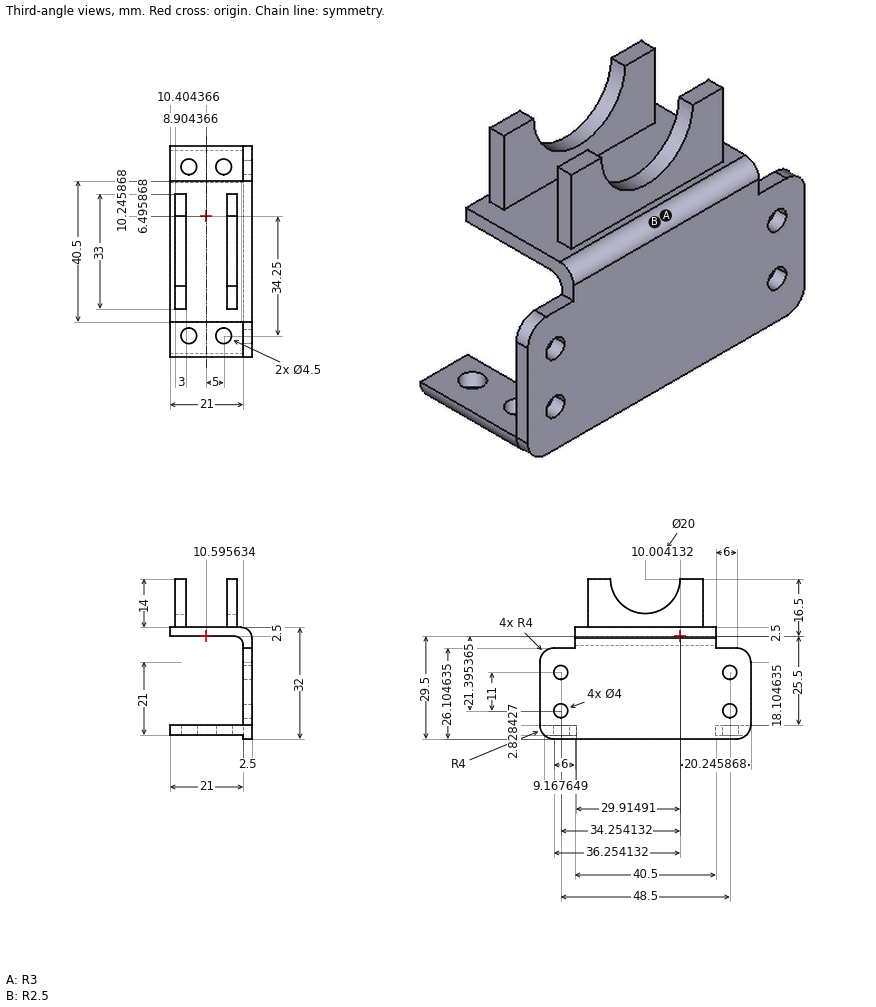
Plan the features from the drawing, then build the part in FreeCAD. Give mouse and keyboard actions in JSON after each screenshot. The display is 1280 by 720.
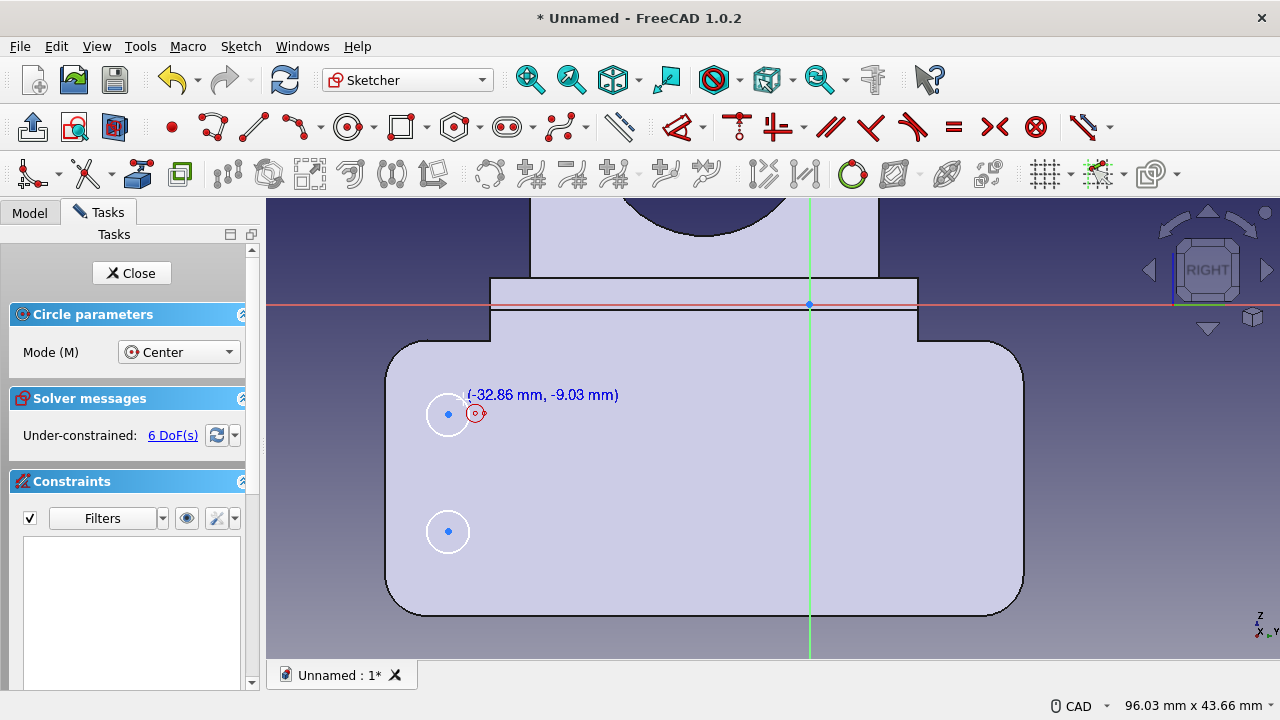
{"action": "left_click", "coordinate": [960, 414]}
{"action": "left_click", "coordinate": [975, 399]}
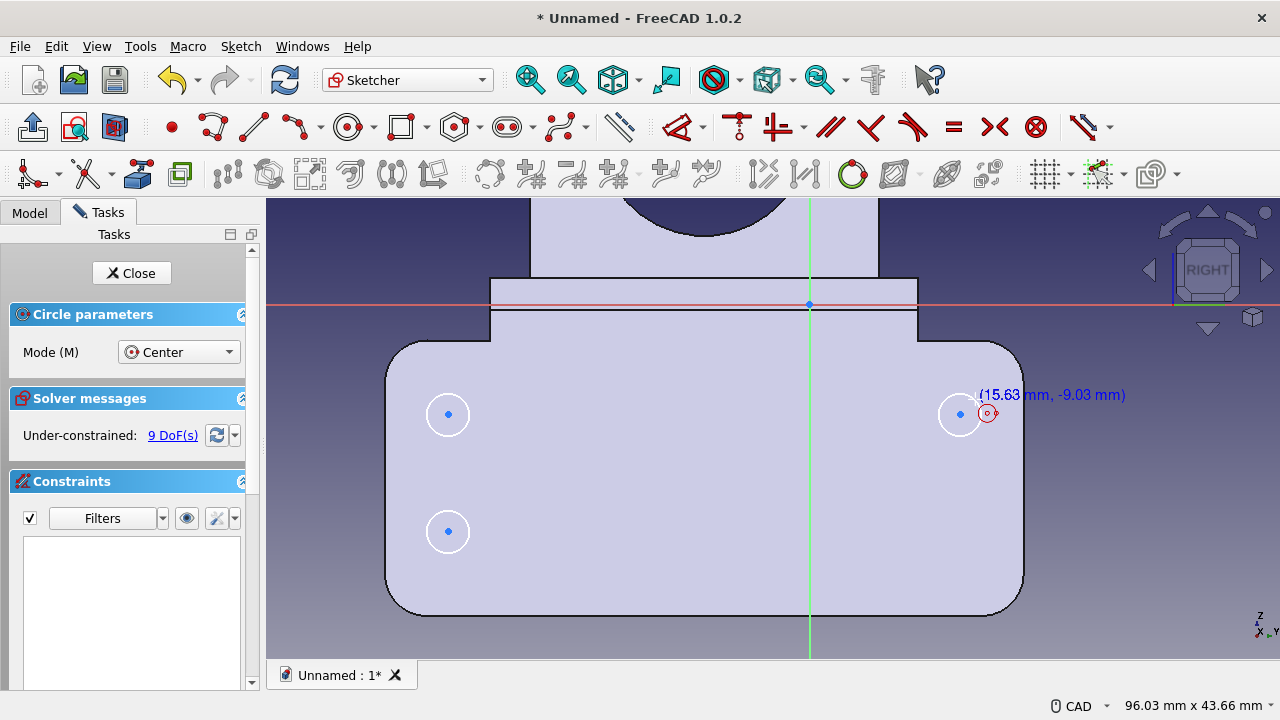
{"action": "left_click", "coordinate": [960, 531]}
{"action": "left_click", "coordinate": [975, 516]}
{"action": "key", "text": "Escape"}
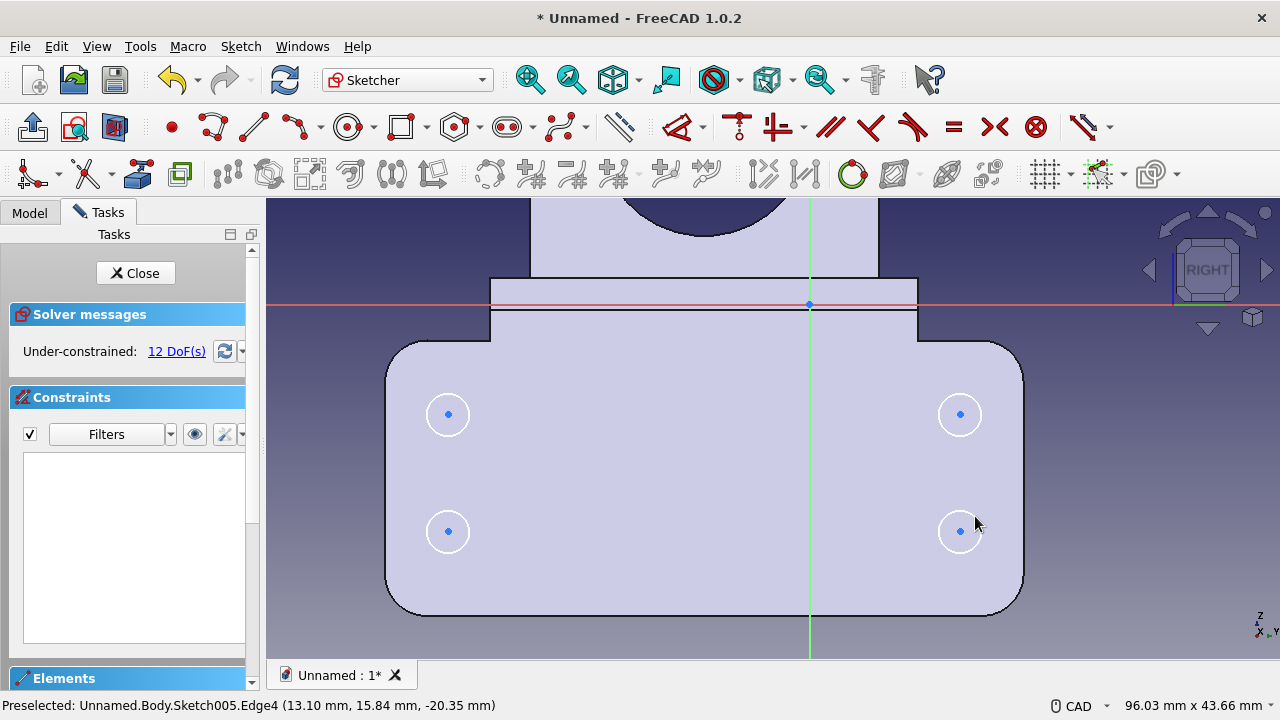
{"action": "left_click", "coordinate": [463, 517]}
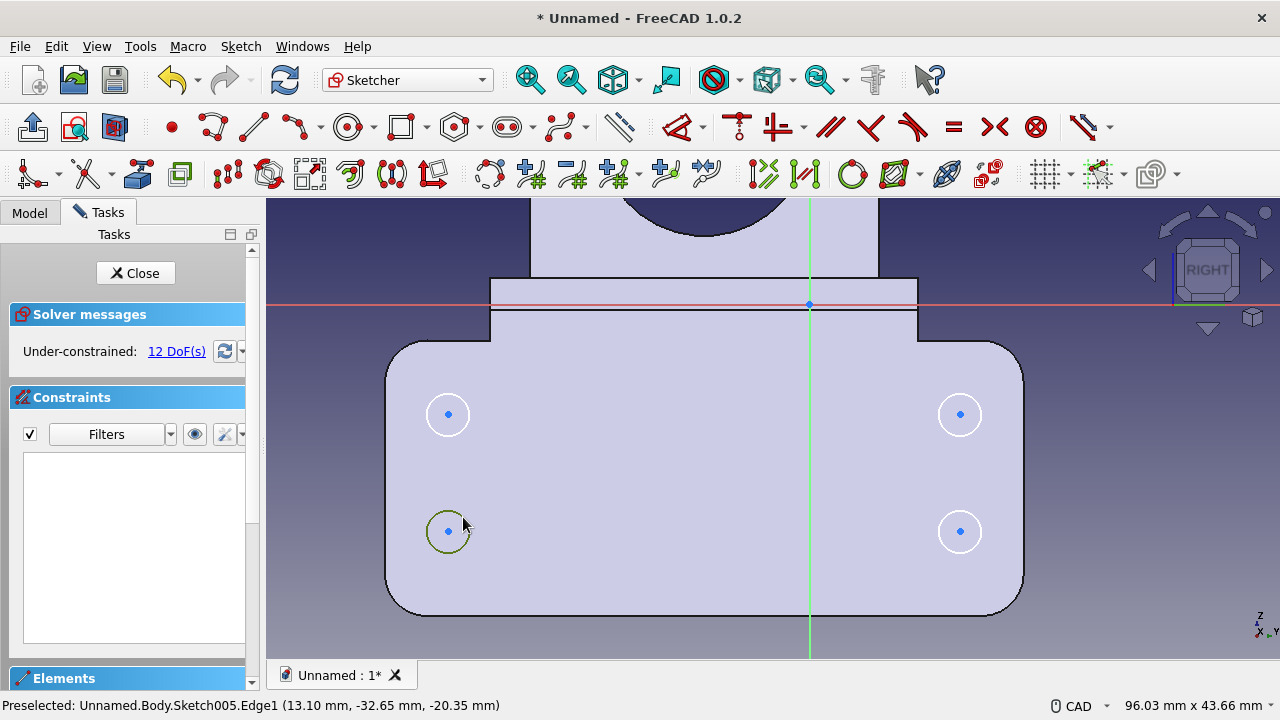
{"action": "left_click", "coordinate": [463, 400]}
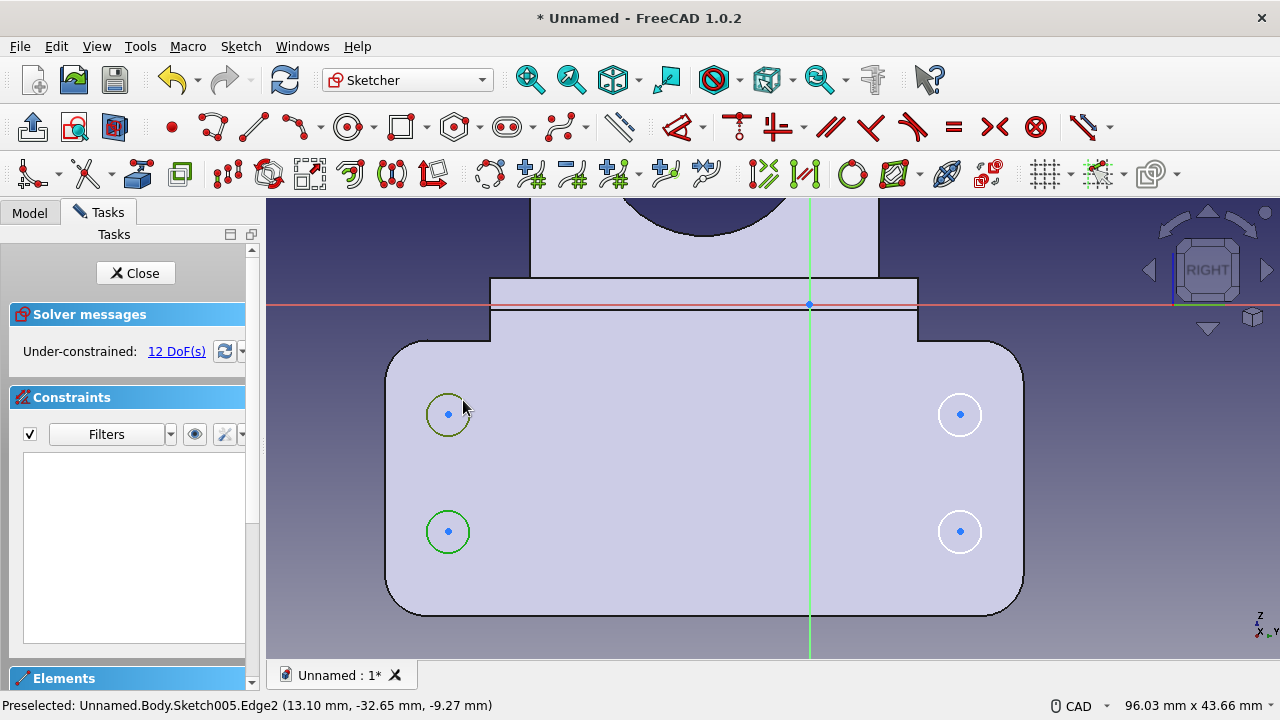
{"action": "left_click", "coordinate": [975, 400]}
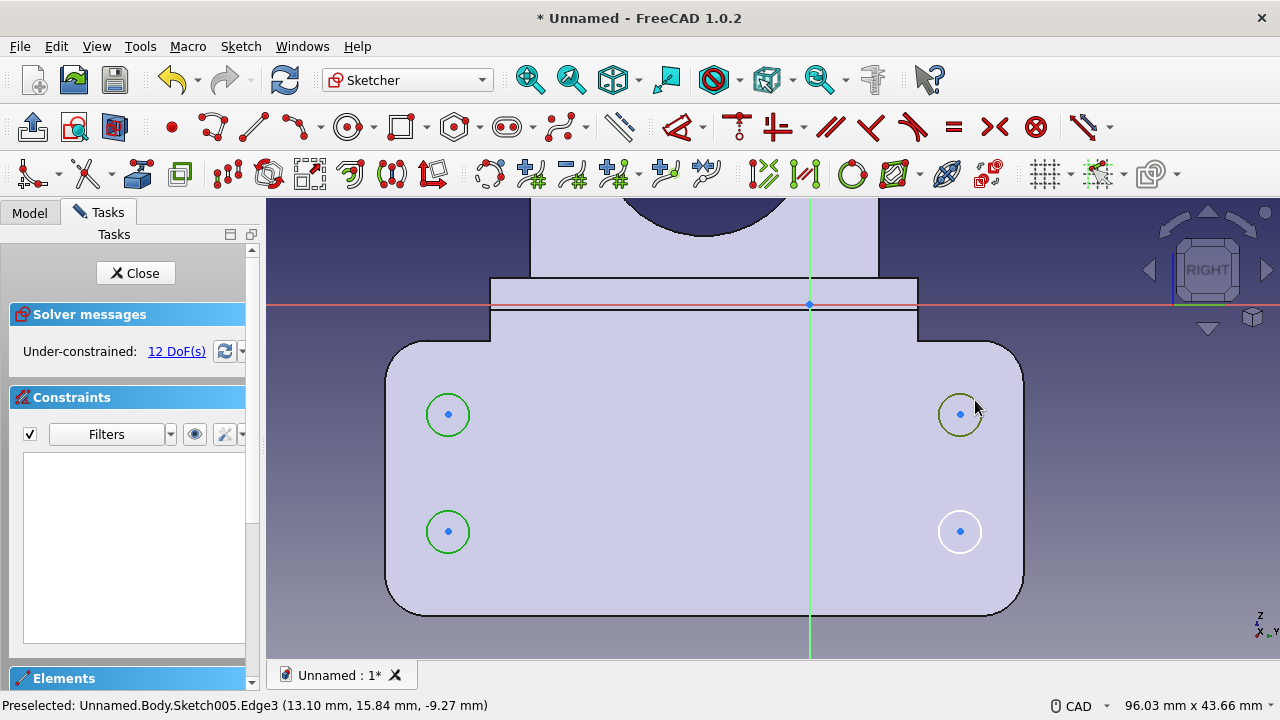
{"action": "left_click", "coordinate": [975, 517]}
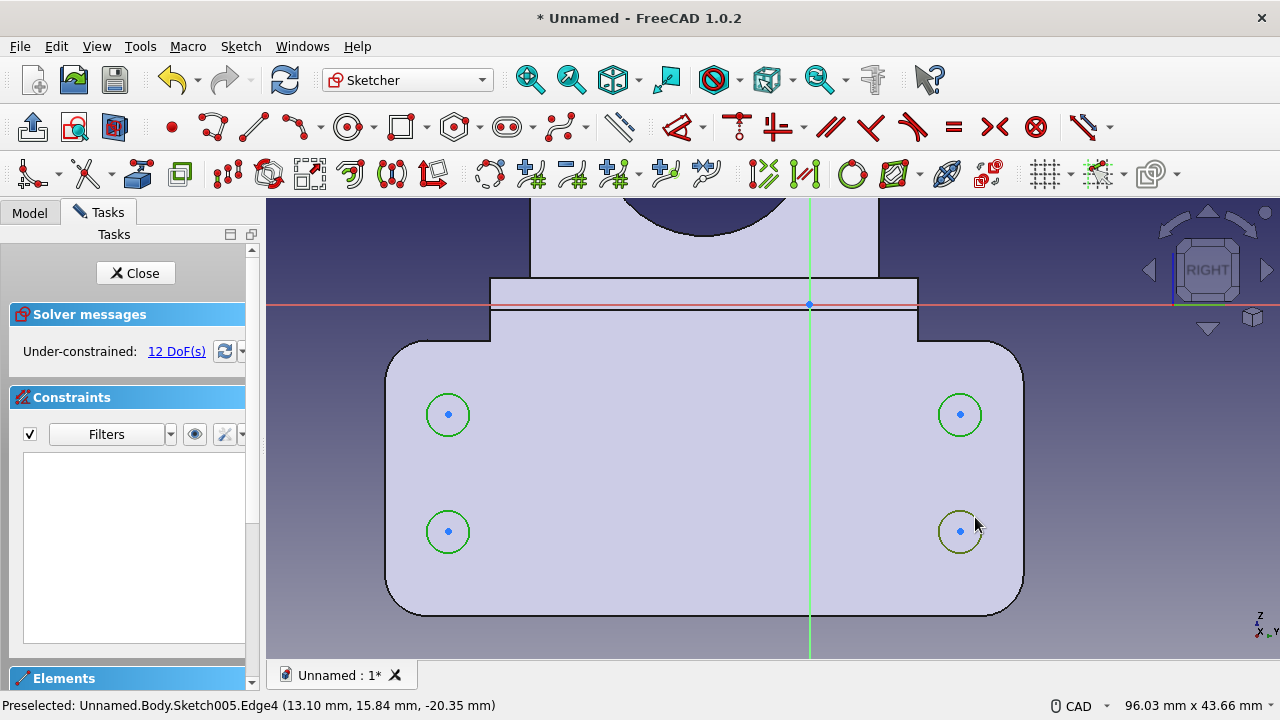
{"action": "left_click", "coordinate": [954, 128]}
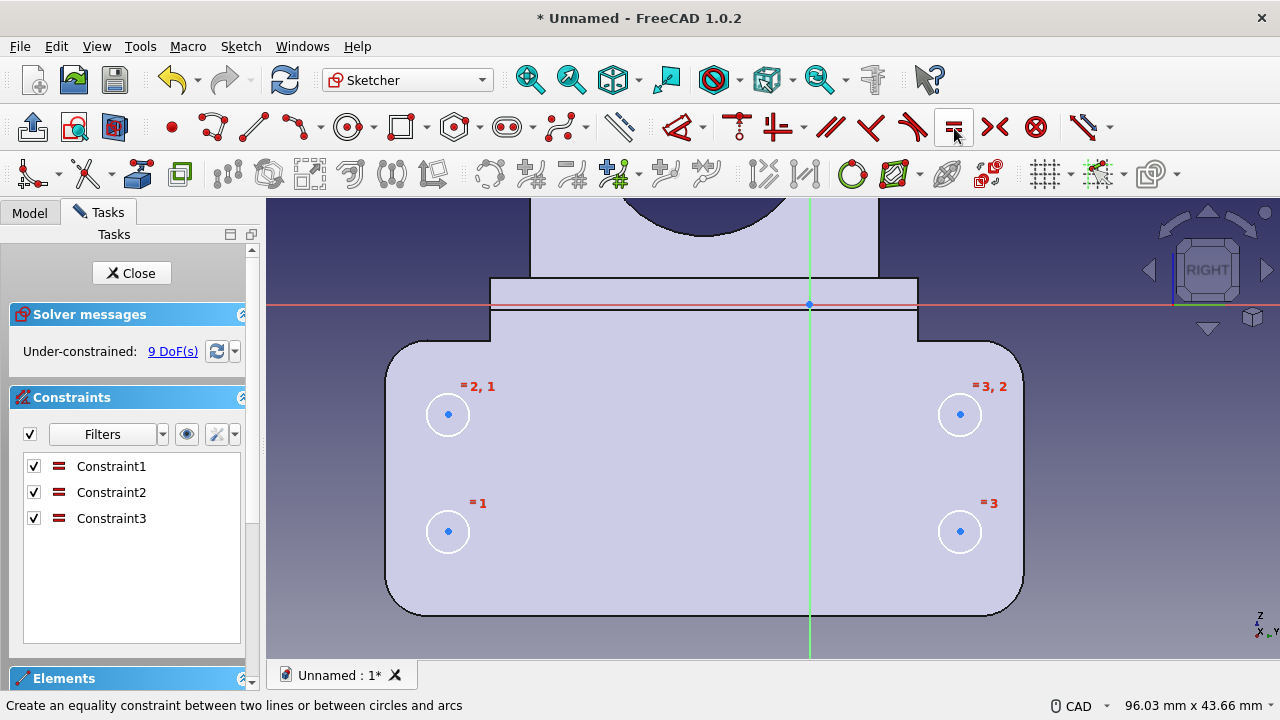
{"action": "left_click", "coordinate": [676, 128]}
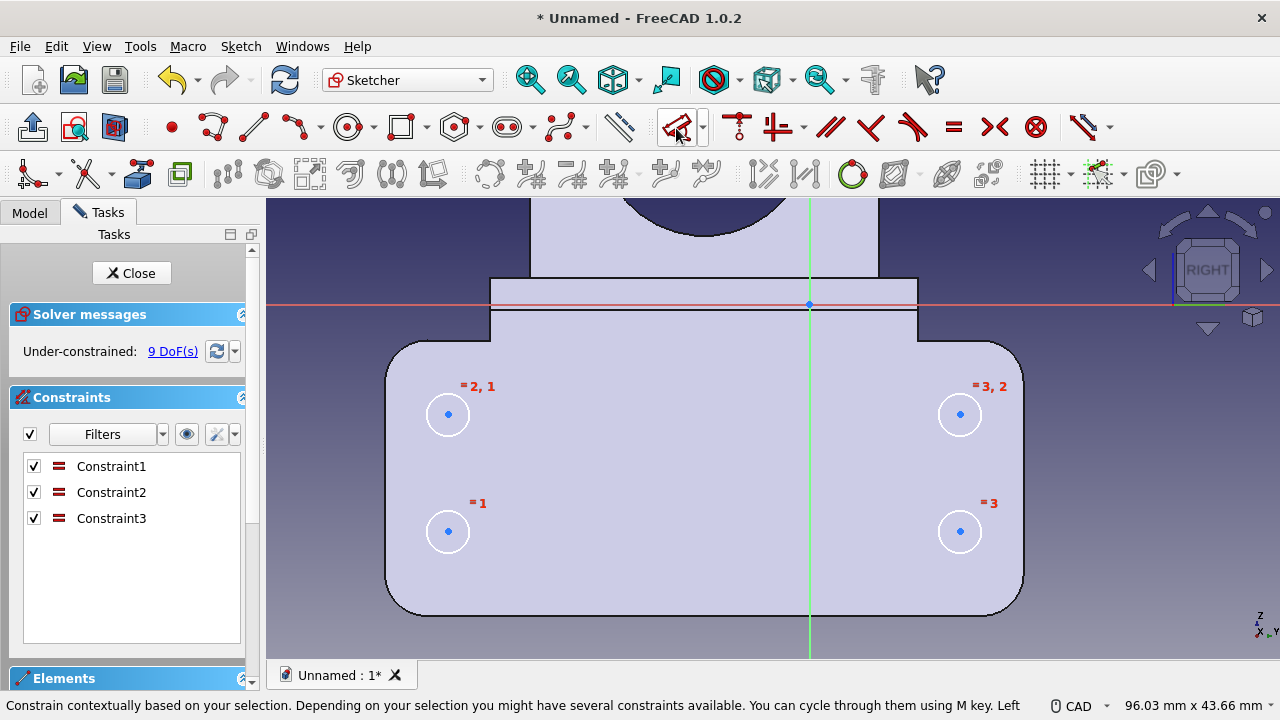
{"action": "left_click", "coordinate": [463, 517]}
{"action": "left_click", "coordinate": [486, 494]}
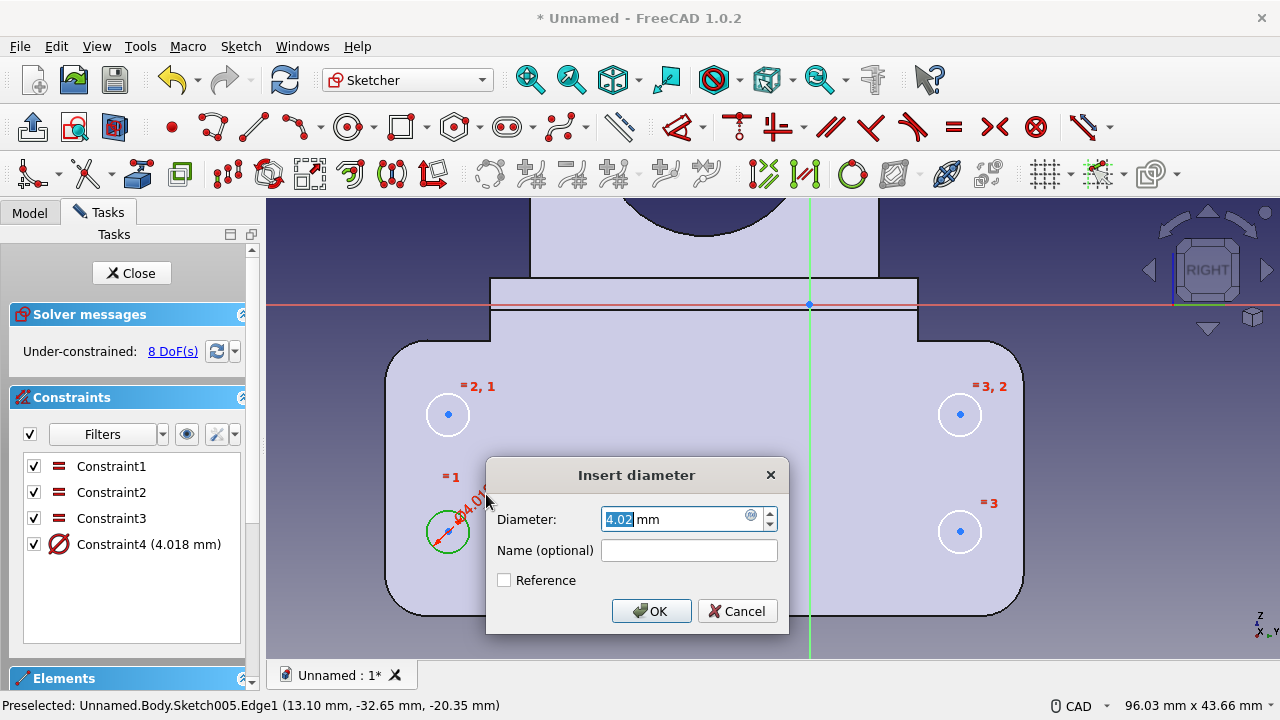
{"action": "type", "text": "4"}
{"action": "key", "text": "Return"}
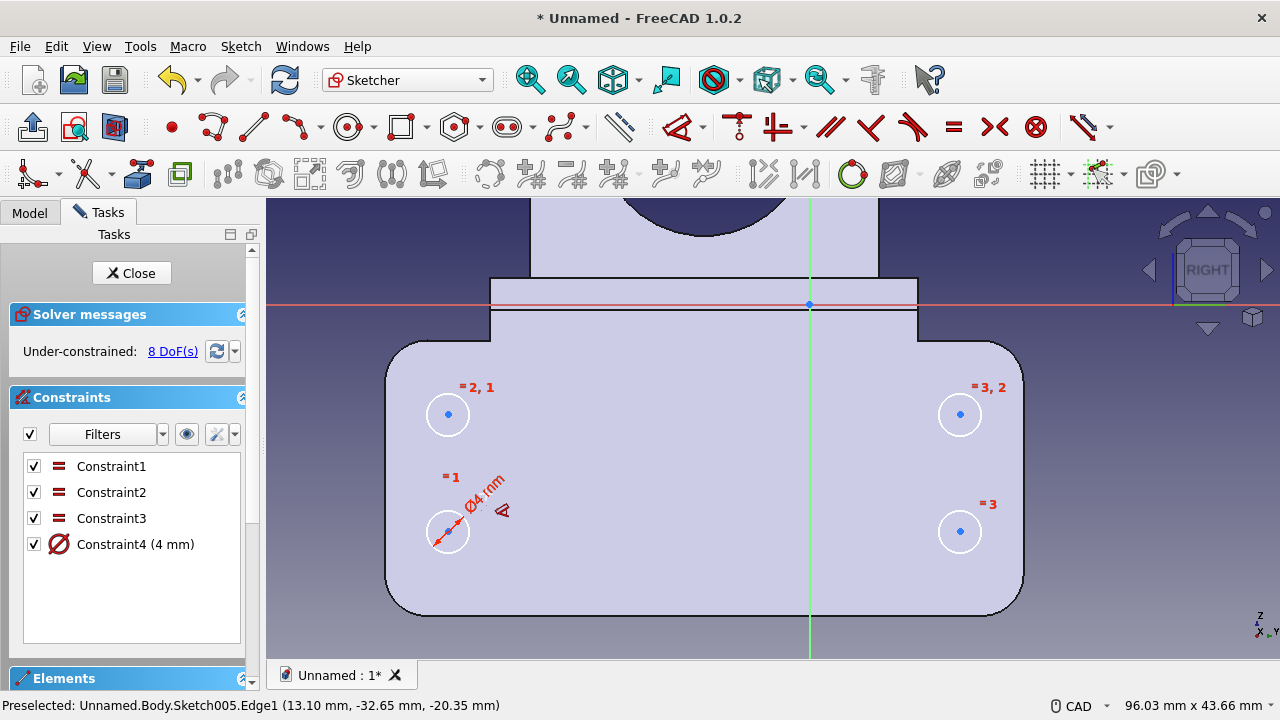
{"action": "left_click", "coordinate": [448, 532]}